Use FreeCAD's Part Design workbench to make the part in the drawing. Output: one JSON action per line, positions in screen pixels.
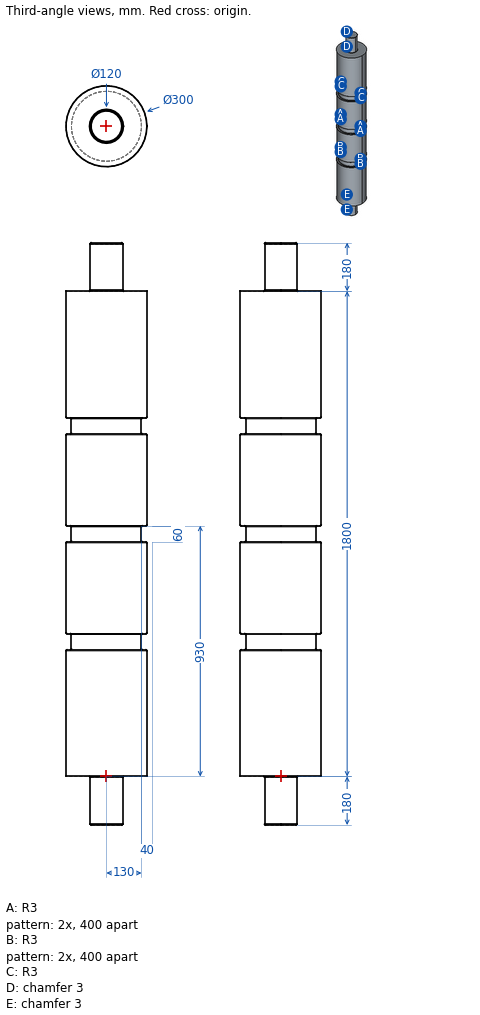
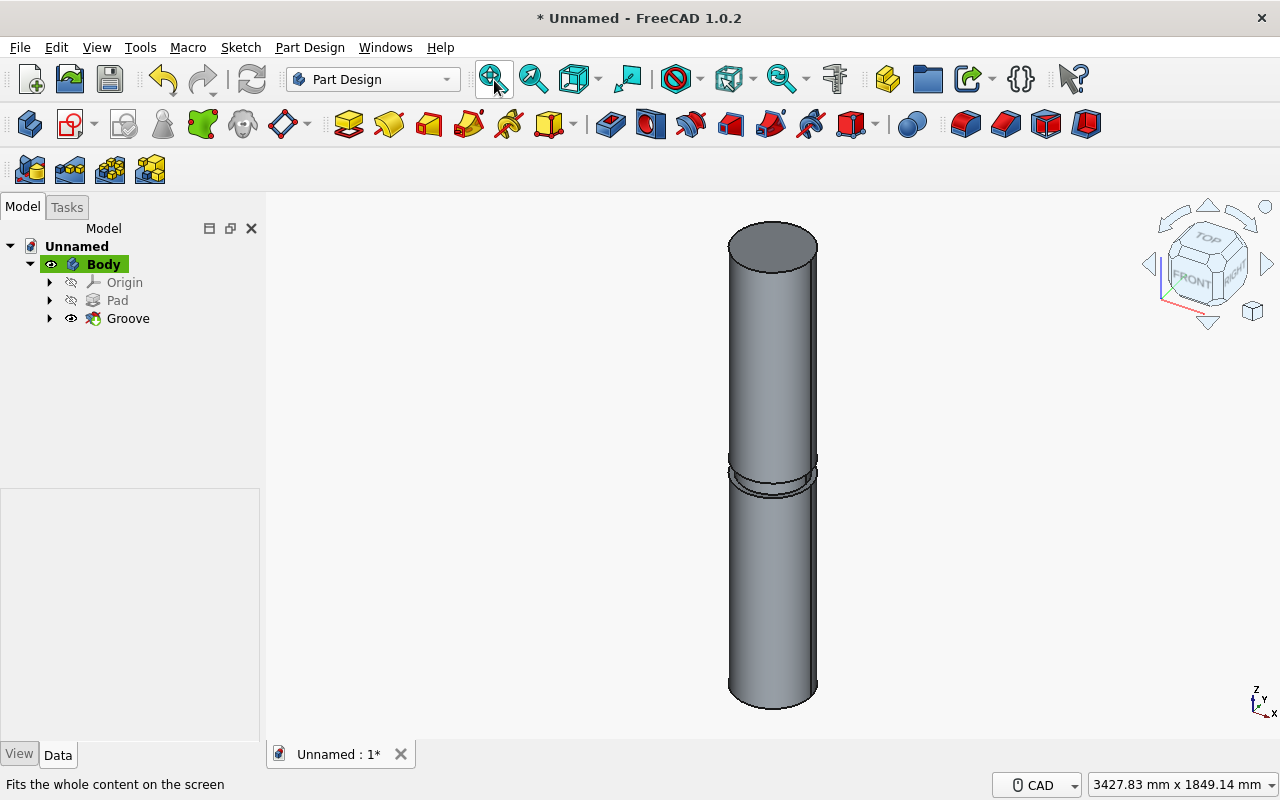
{"action": "left_click", "coordinate": [786, 482]}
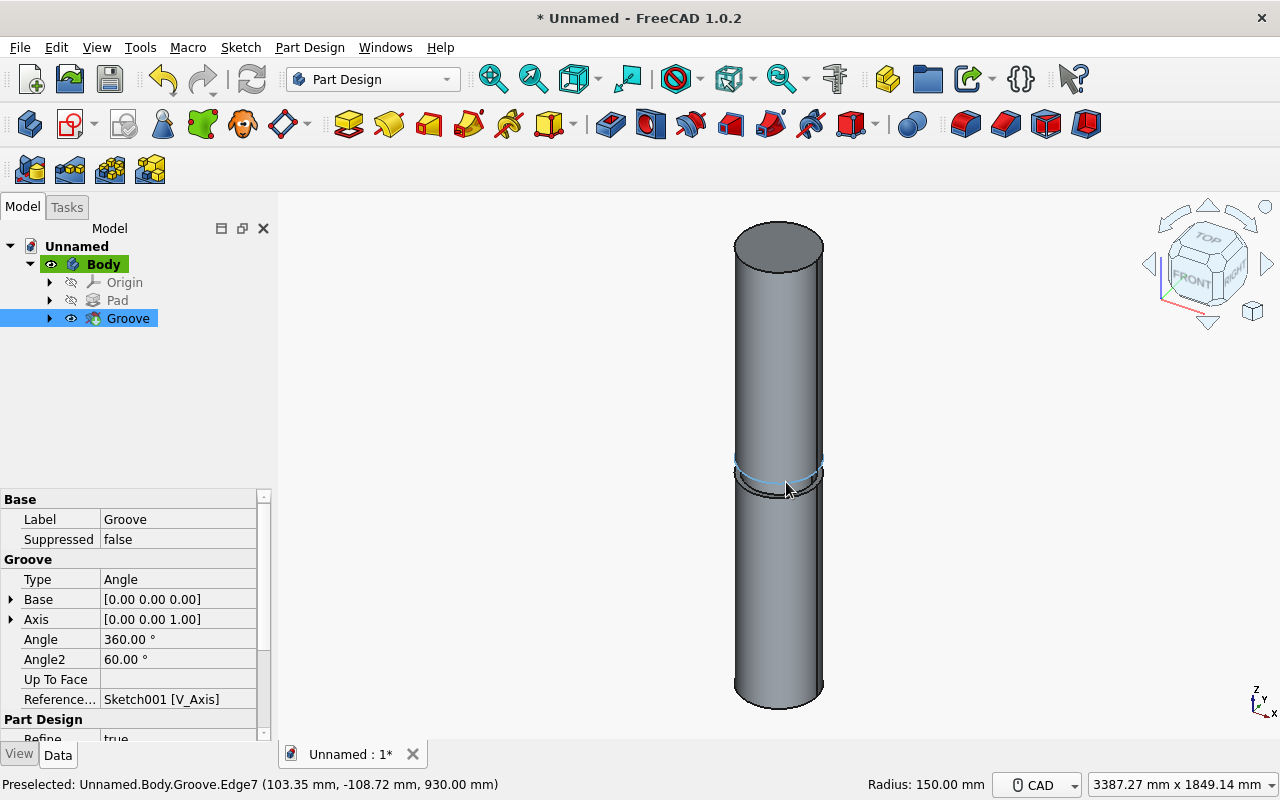
{"action": "left_click", "coordinate": [735, 474], "text": "ctrl"}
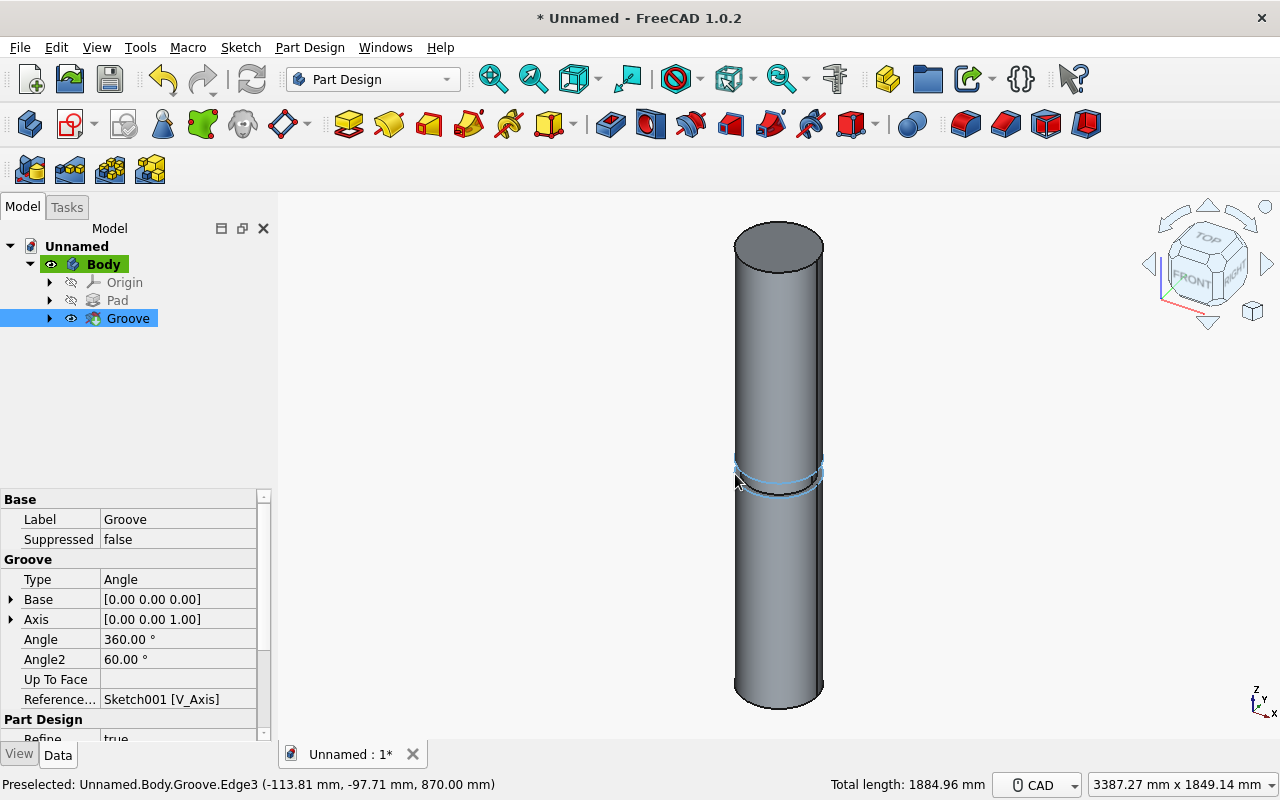
{"action": "key", "text": "0"}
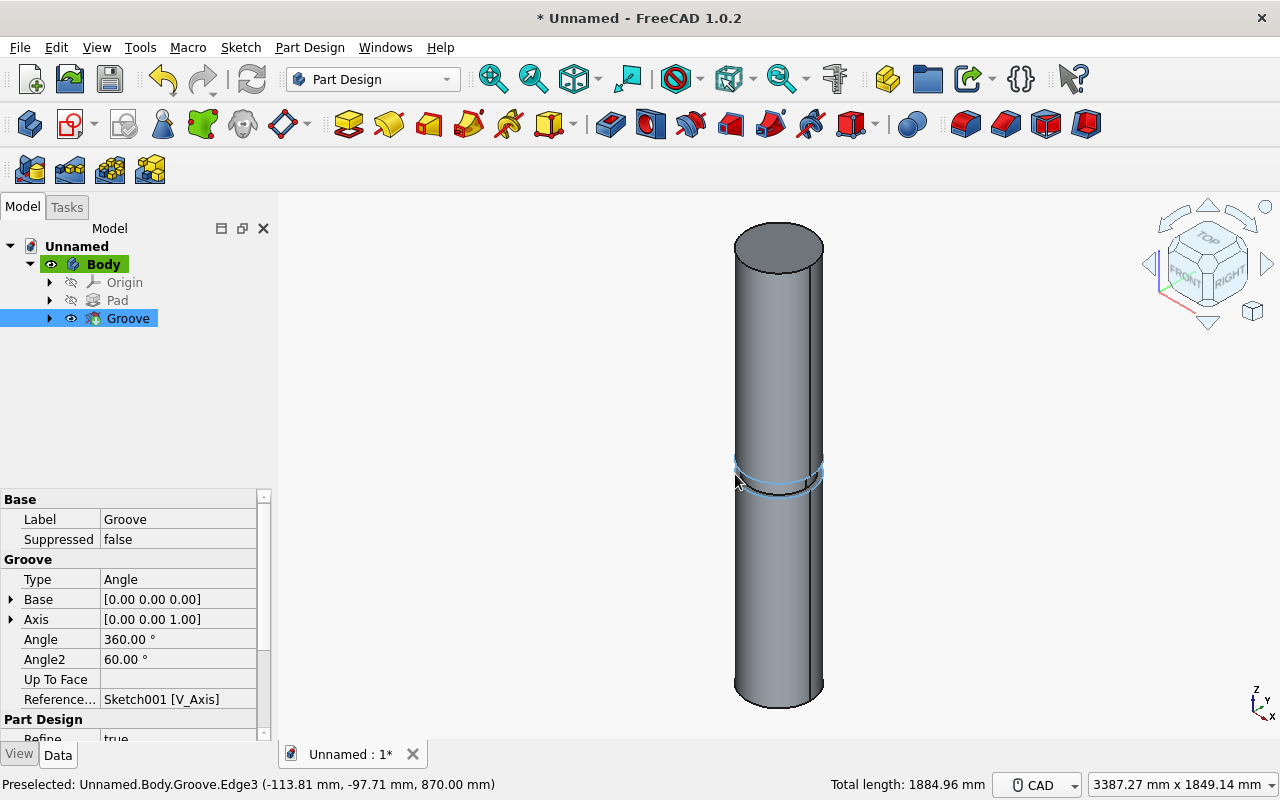
{"action": "key", "text": "2"}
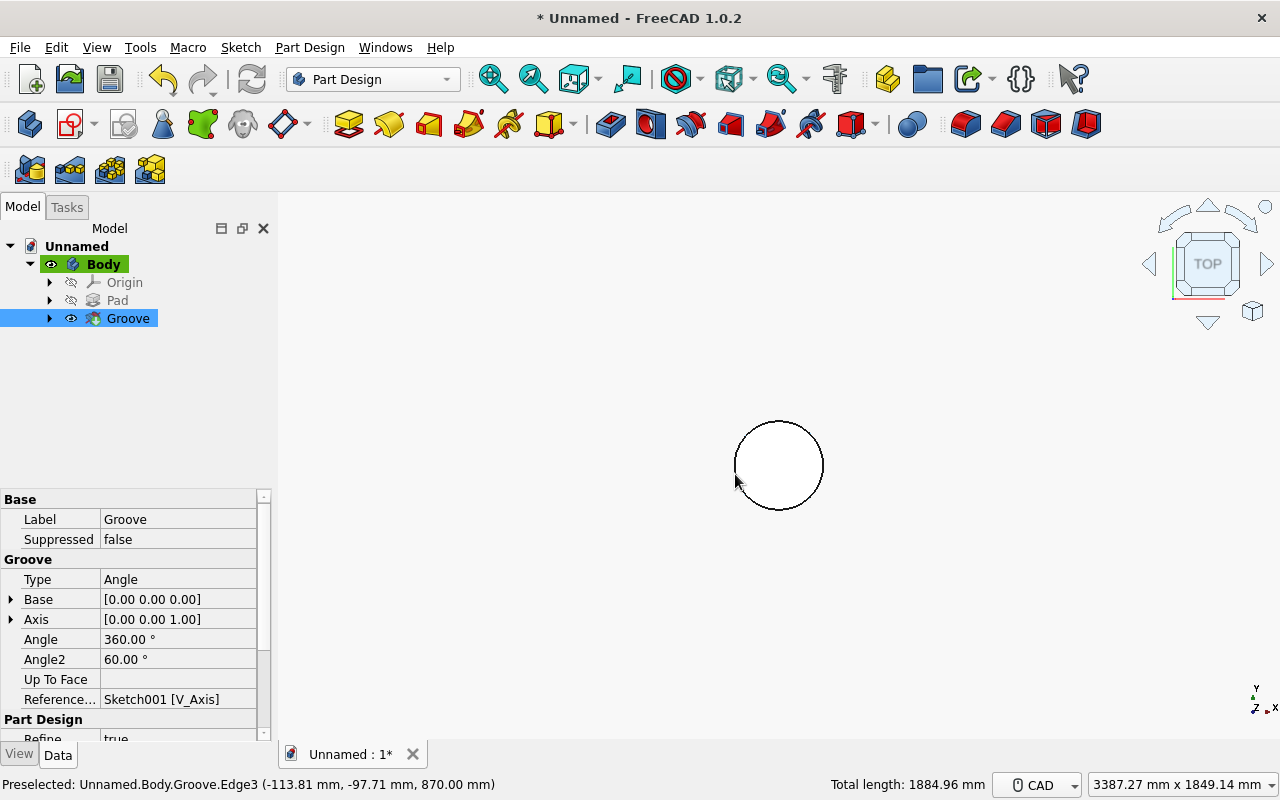
{"action": "key", "text": "v f"}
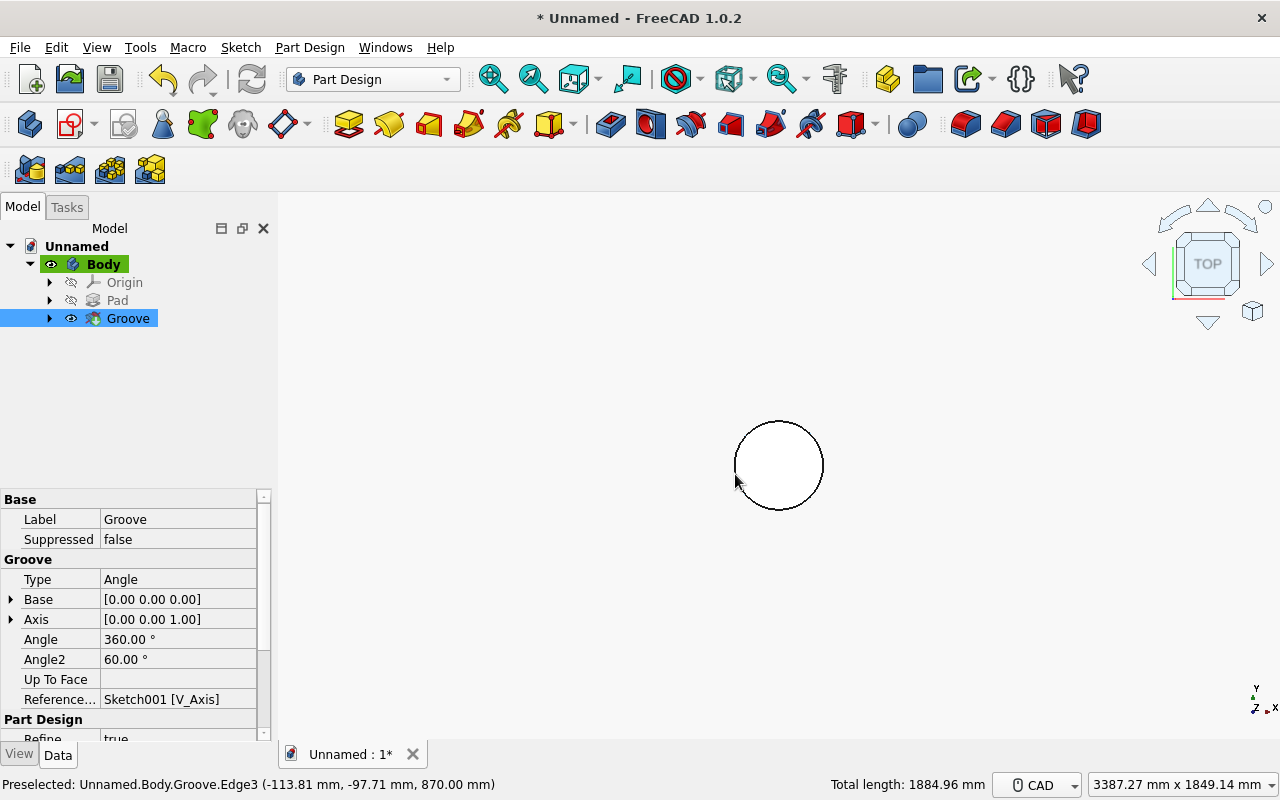
{"action": "key", "text": "1"}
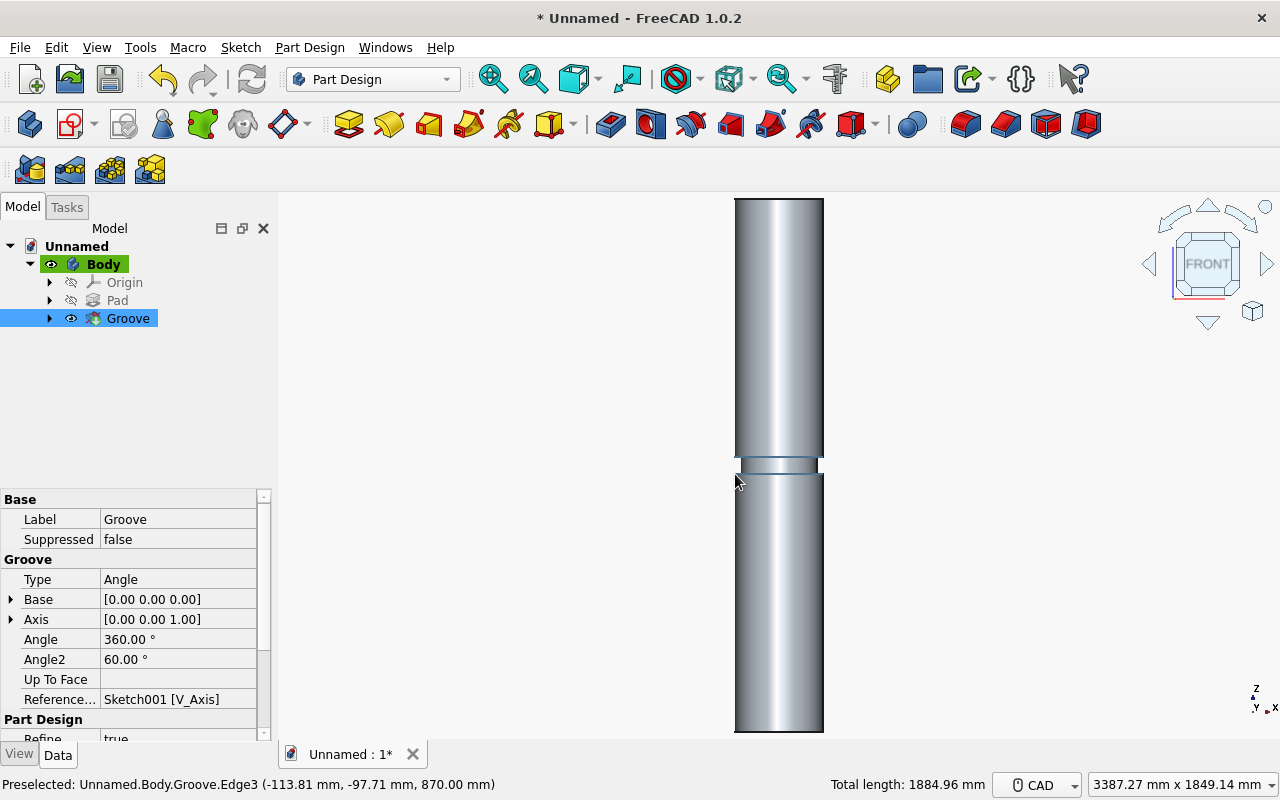
{"action": "key", "text": "3"}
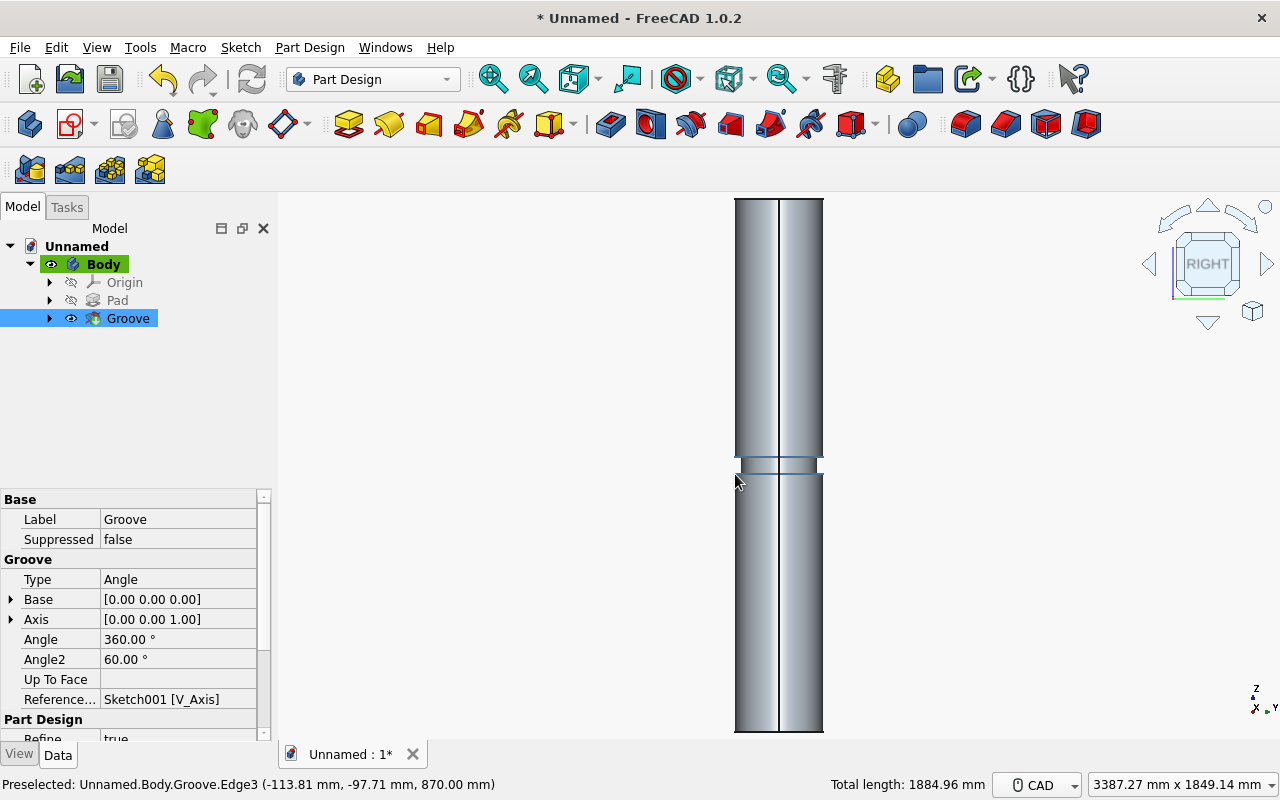
{"action": "key", "text": "5"}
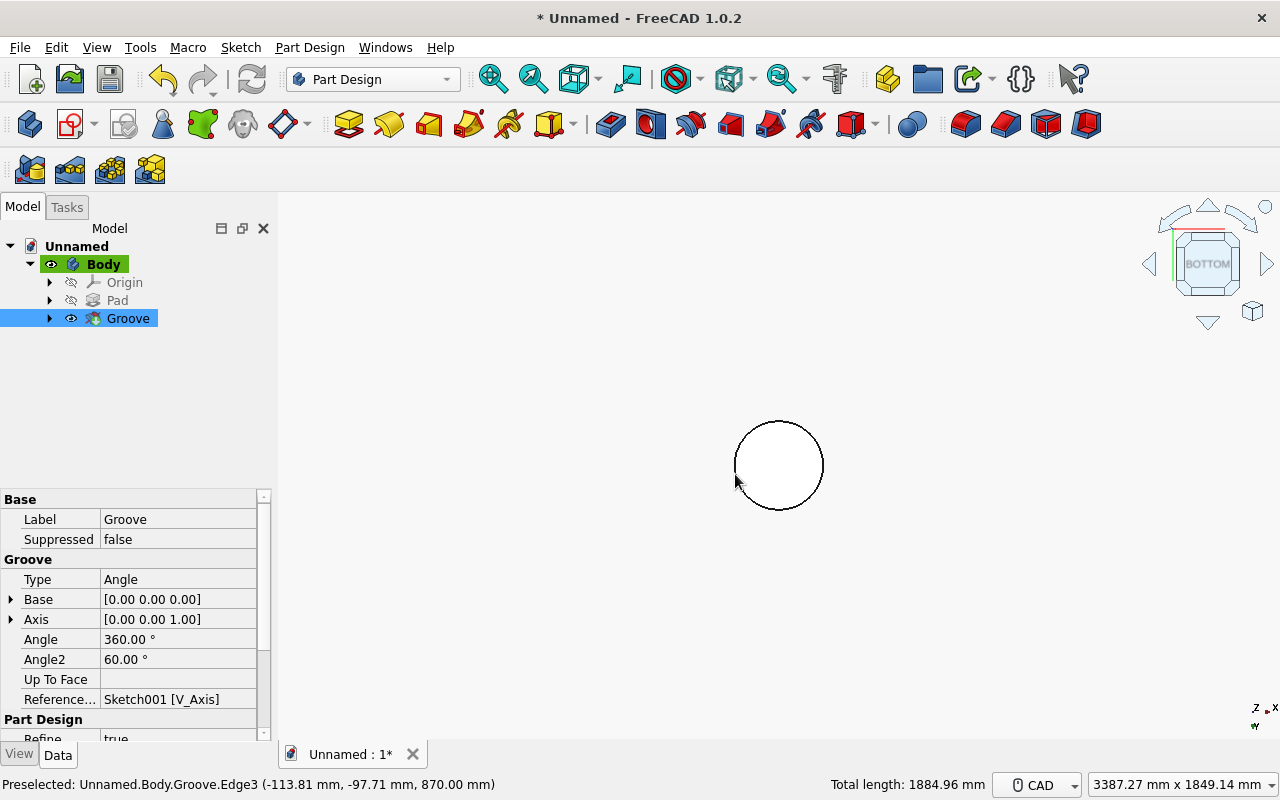
{"action": "left_click", "coordinate": [494, 80]}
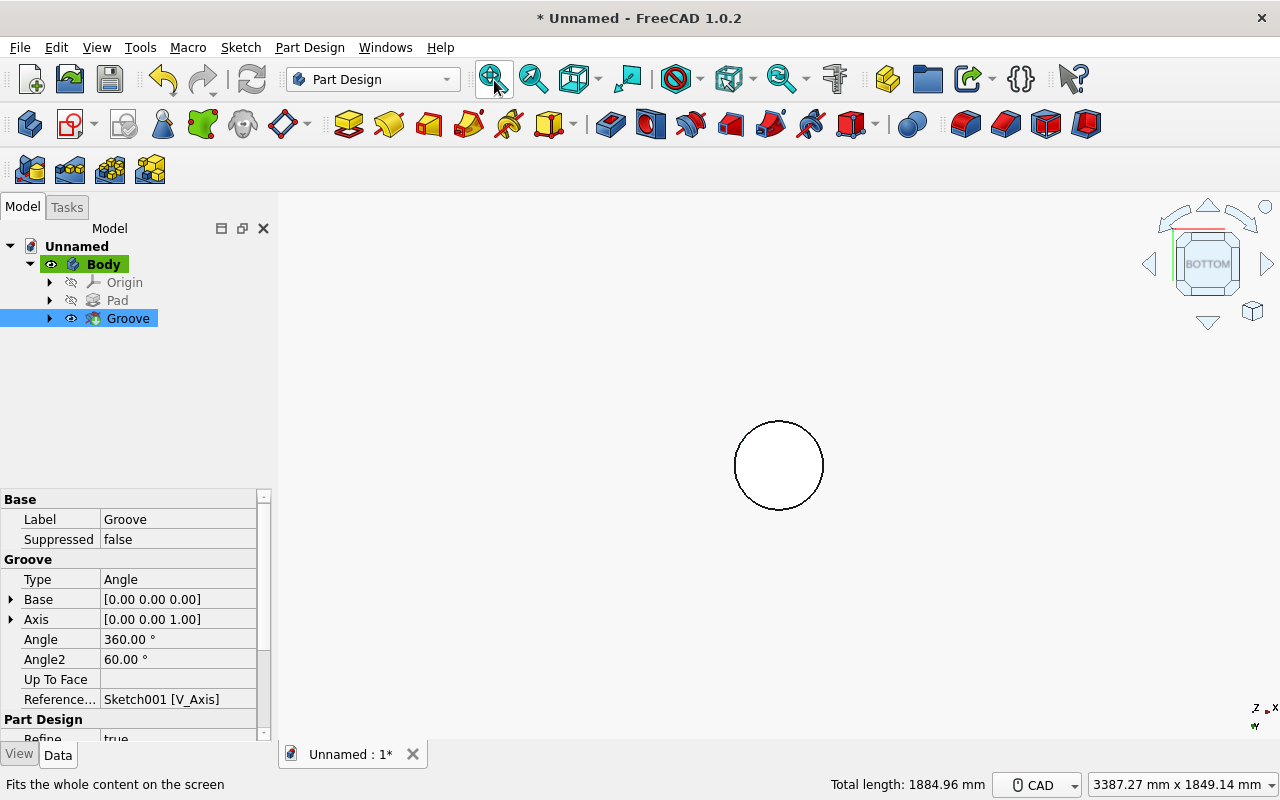
{"action": "key", "text": "4"}